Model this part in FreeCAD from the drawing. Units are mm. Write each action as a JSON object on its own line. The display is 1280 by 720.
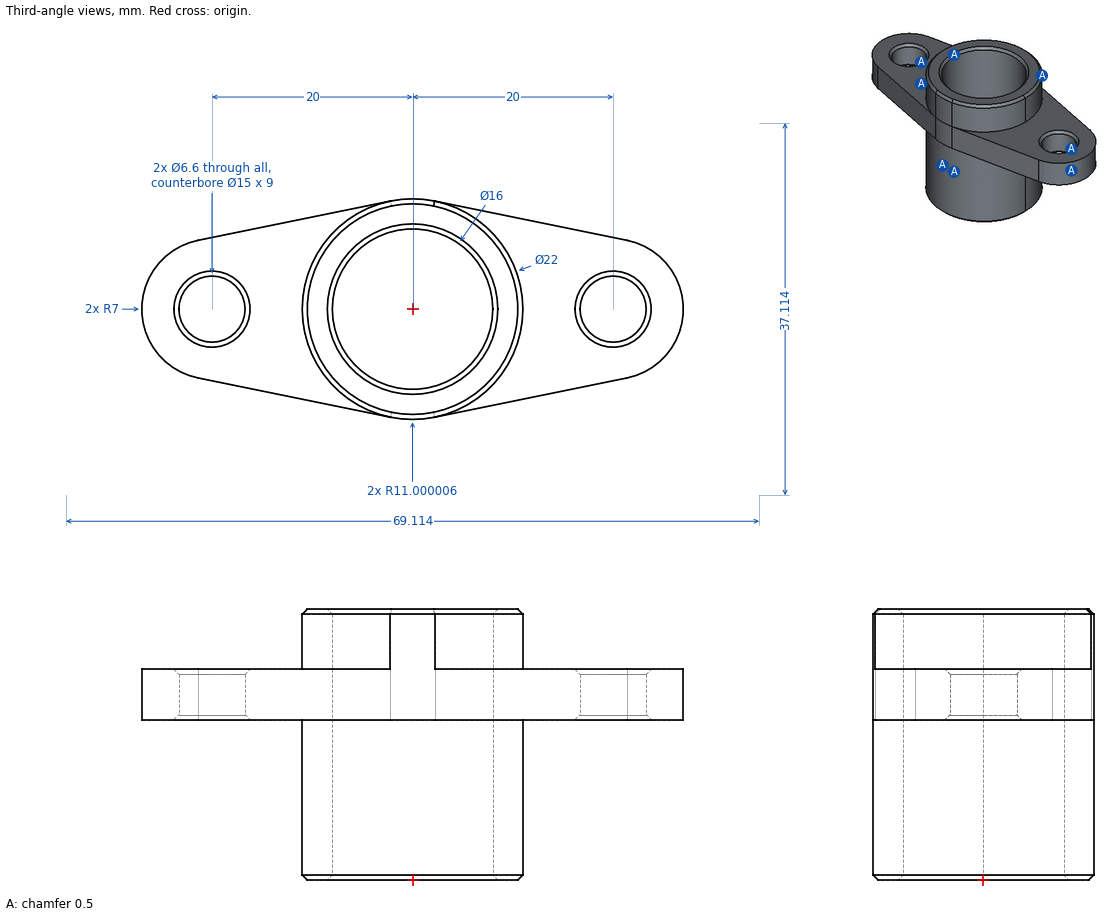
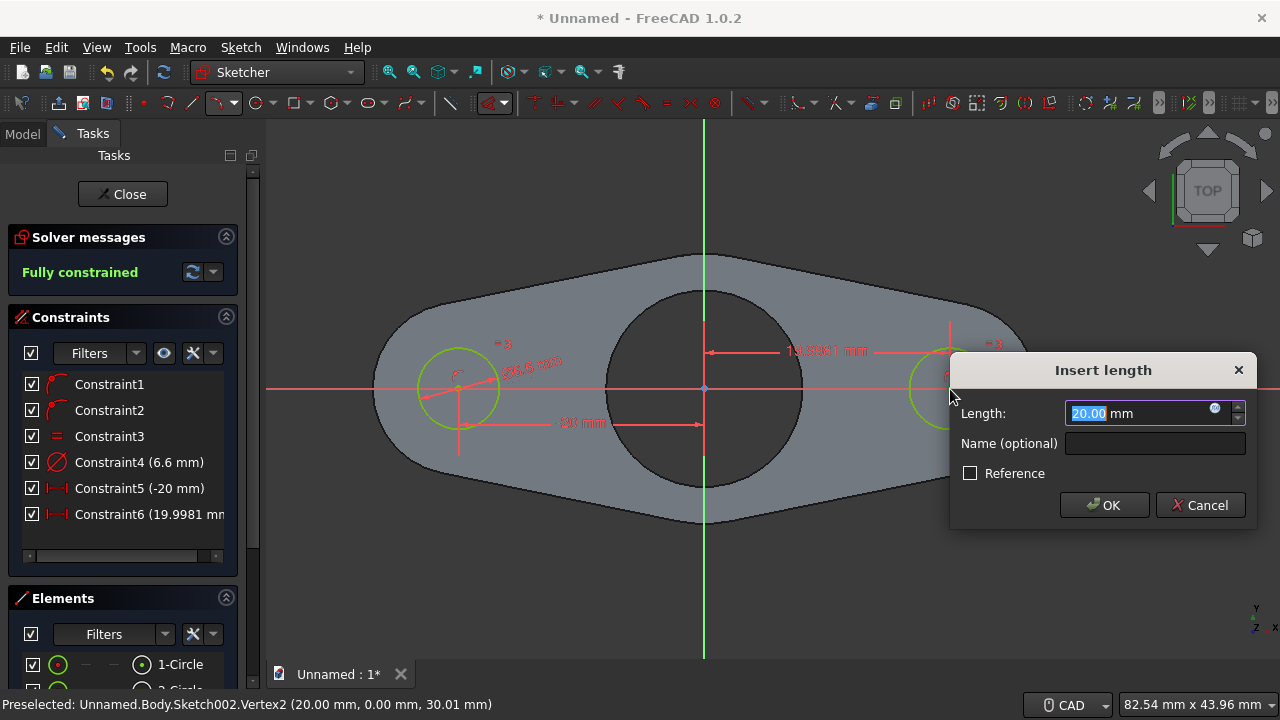
{"action": "type", "text": "20"}
{"action": "key", "text": "Return"}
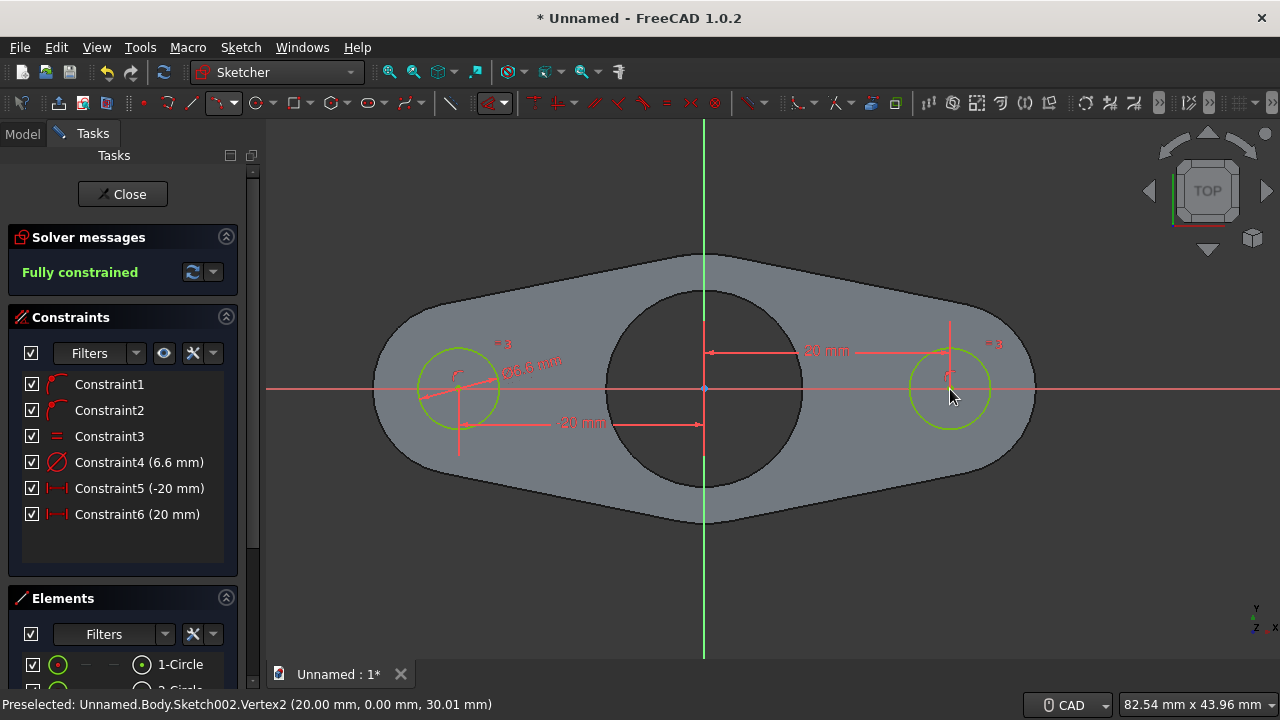
{"action": "left_click", "coordinate": [123, 194]}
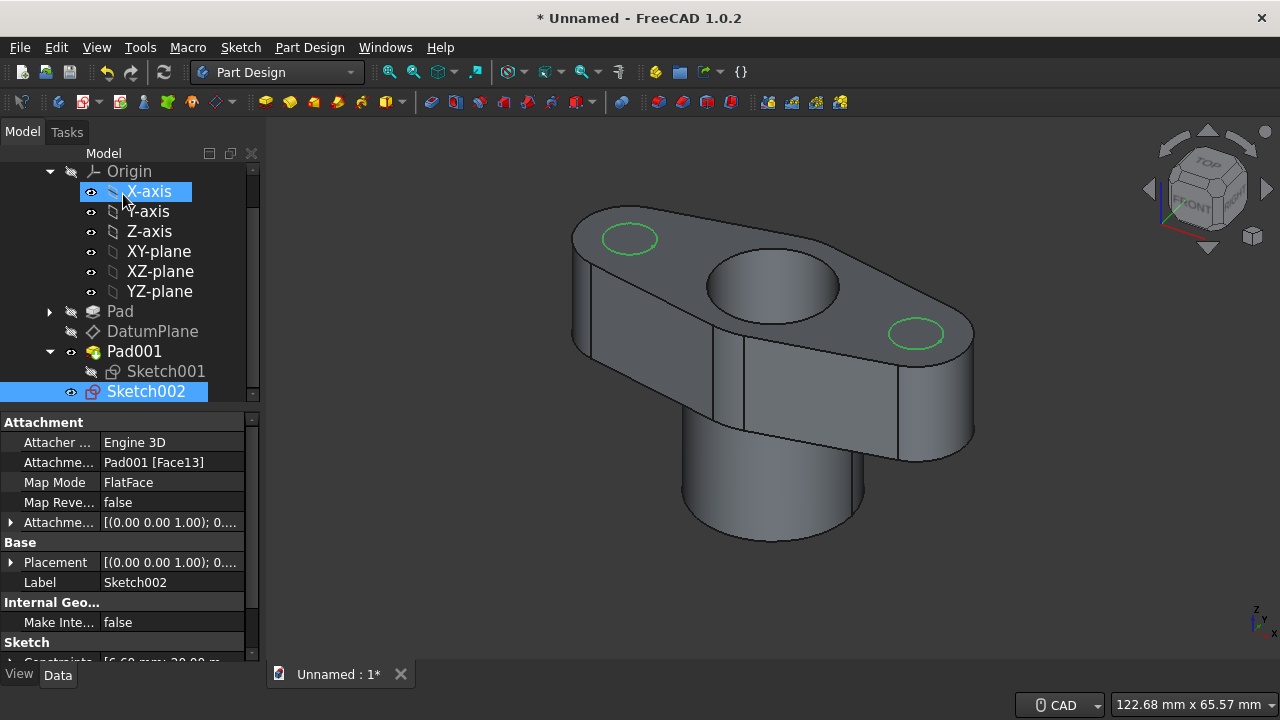
{"action": "left_click", "coordinate": [456, 102]}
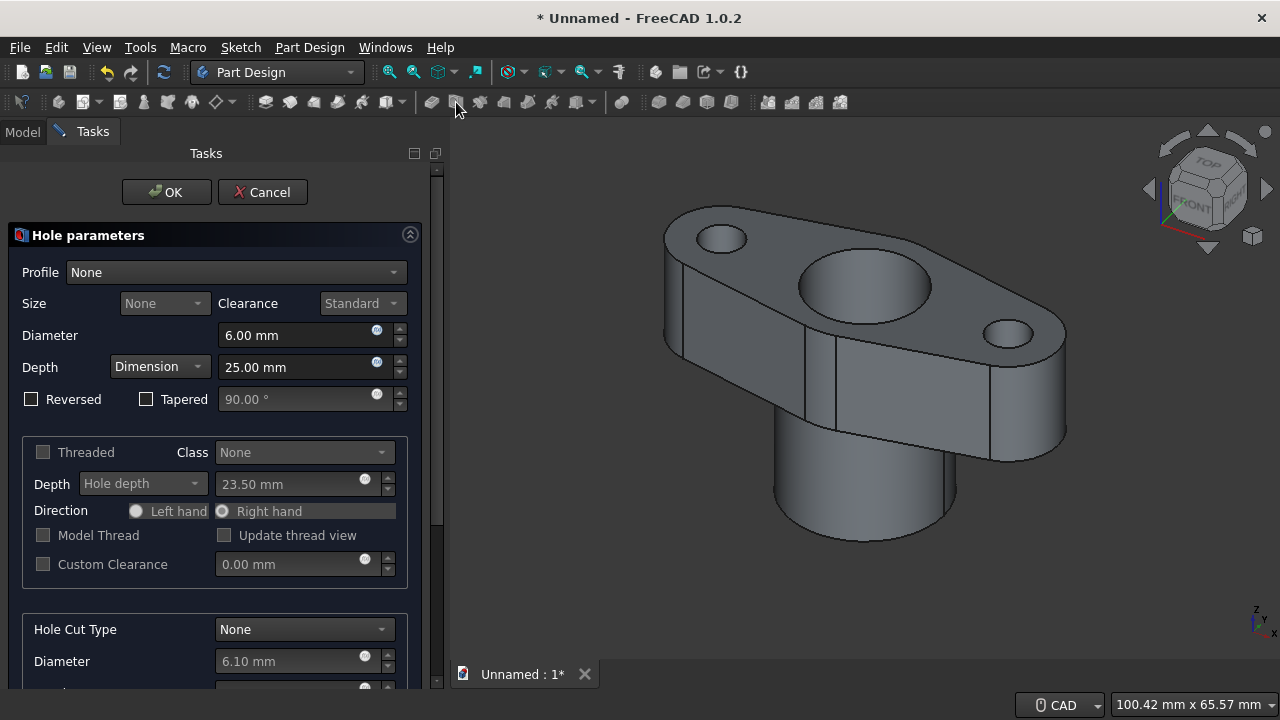
{"action": "triple_click", "coordinate": [305, 335]}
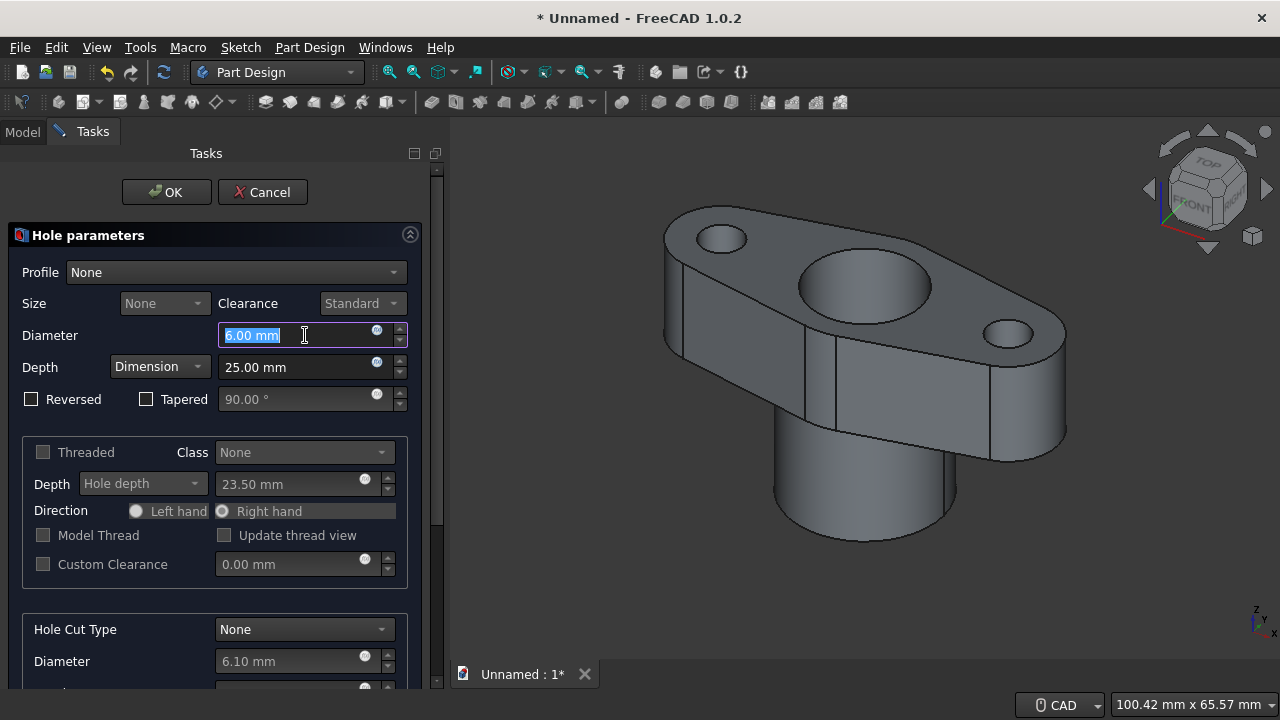
{"action": "type", "text": "6.6"}
{"action": "key", "text": "Tab"}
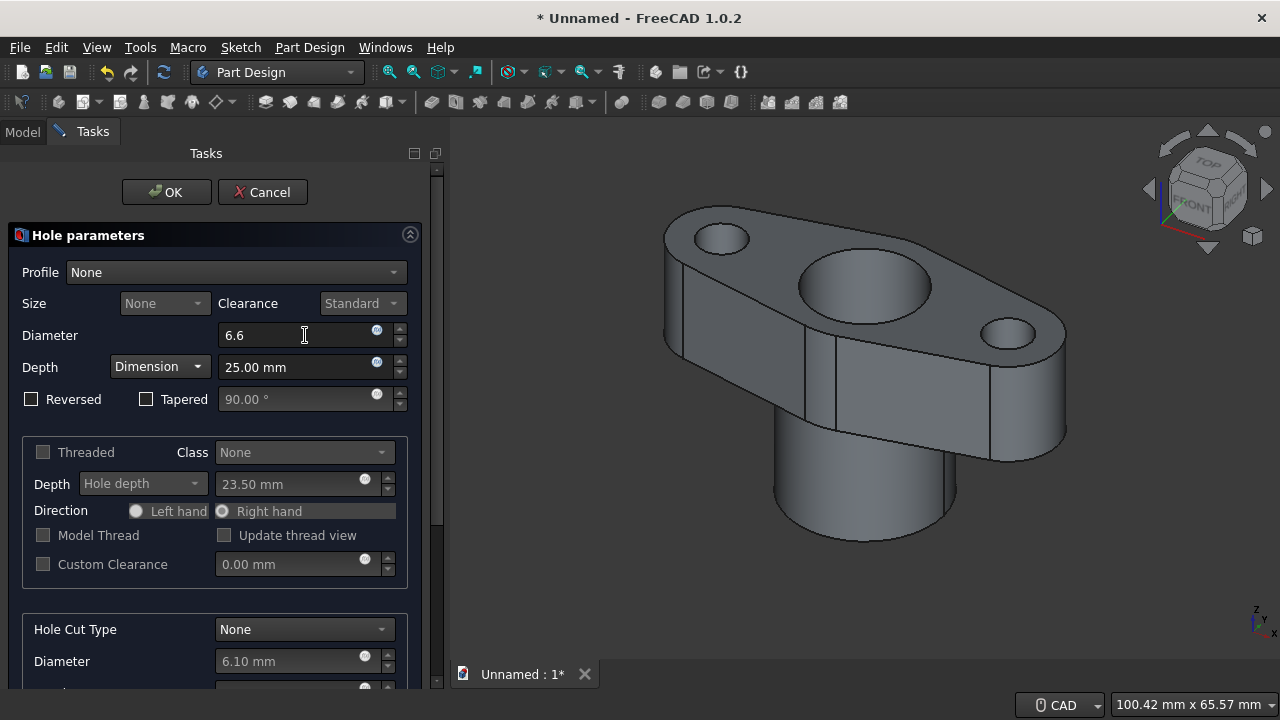
{"action": "left_click", "coordinate": [161, 366]}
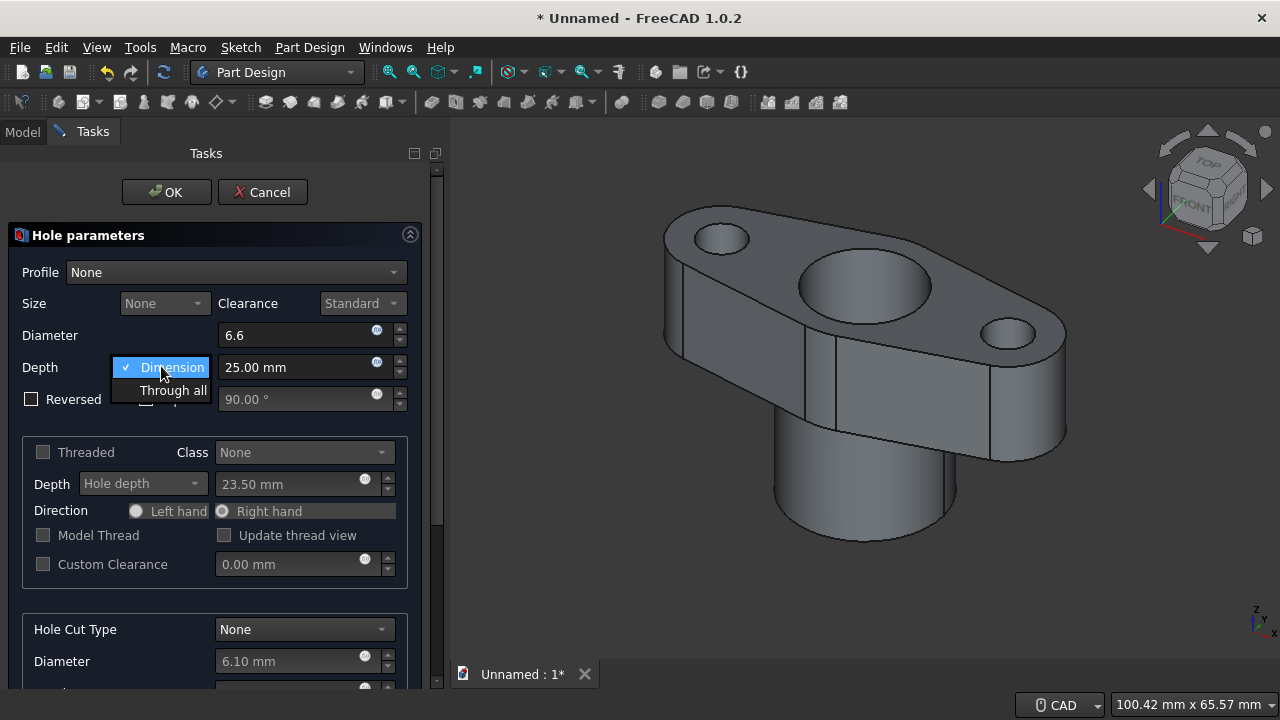
{"action": "left_click", "coordinate": [160, 390]}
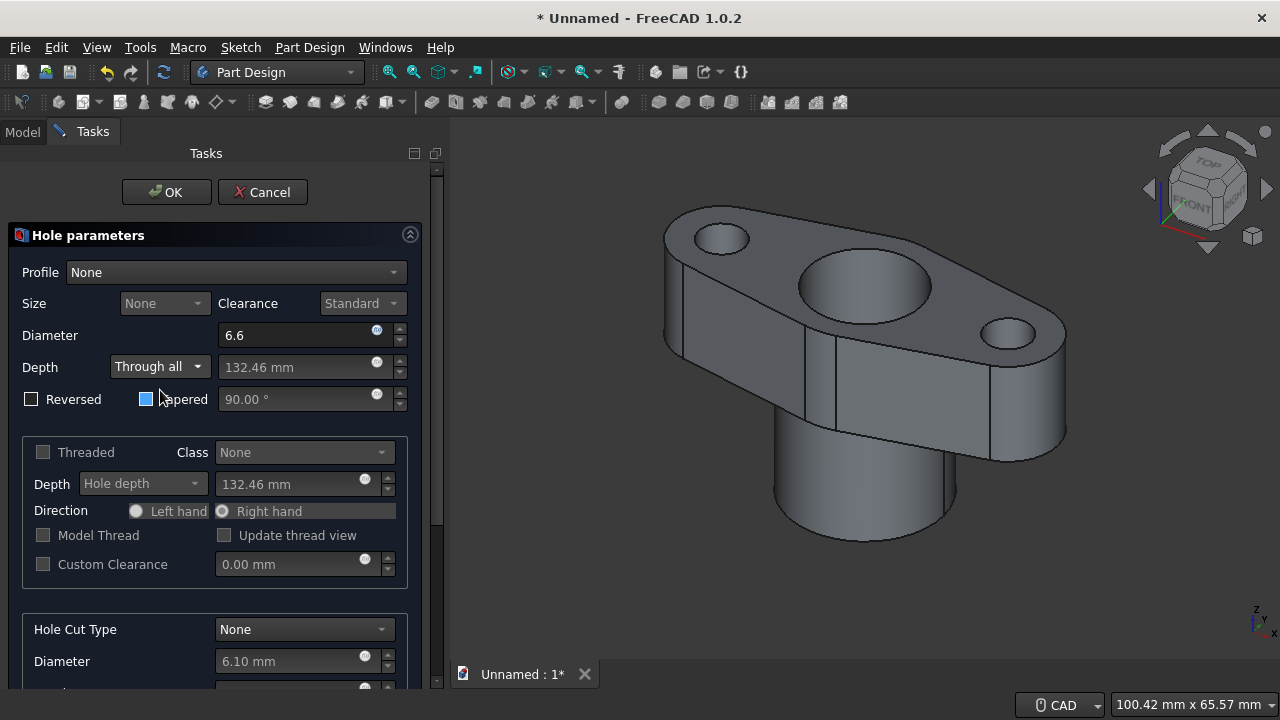
{"action": "left_click", "coordinate": [306, 630]}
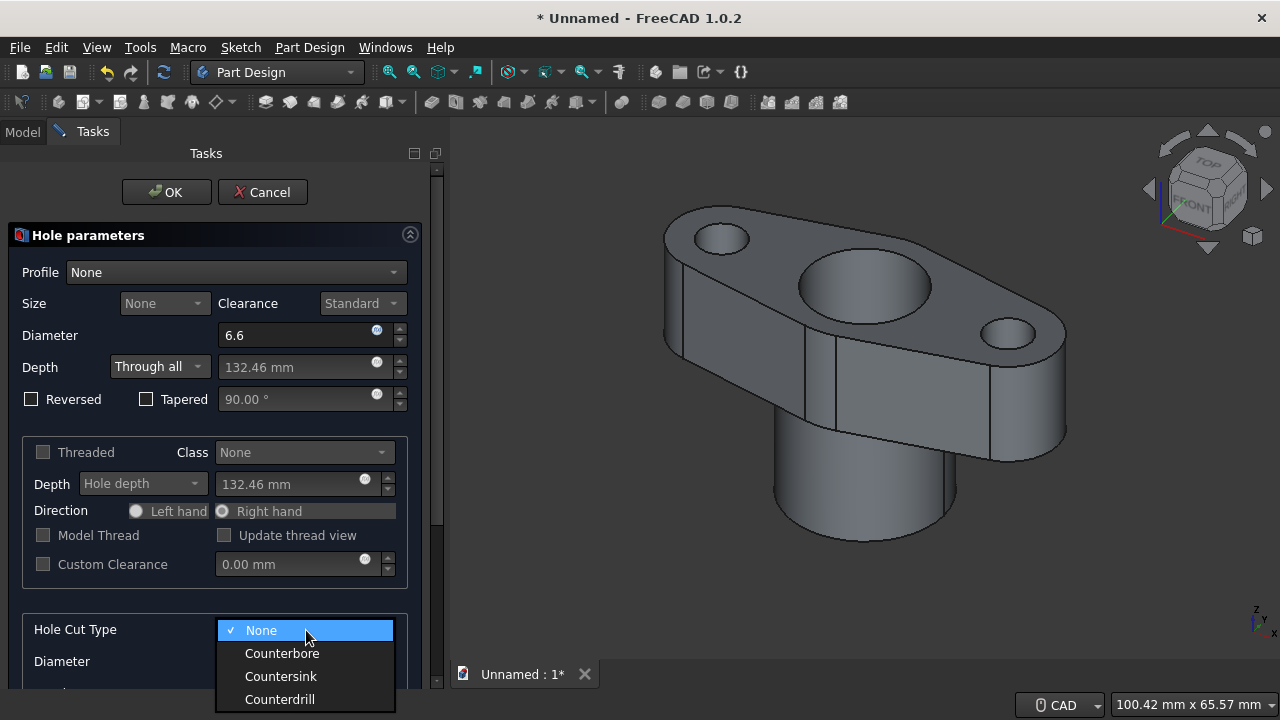
{"action": "left_click", "coordinate": [304, 654]}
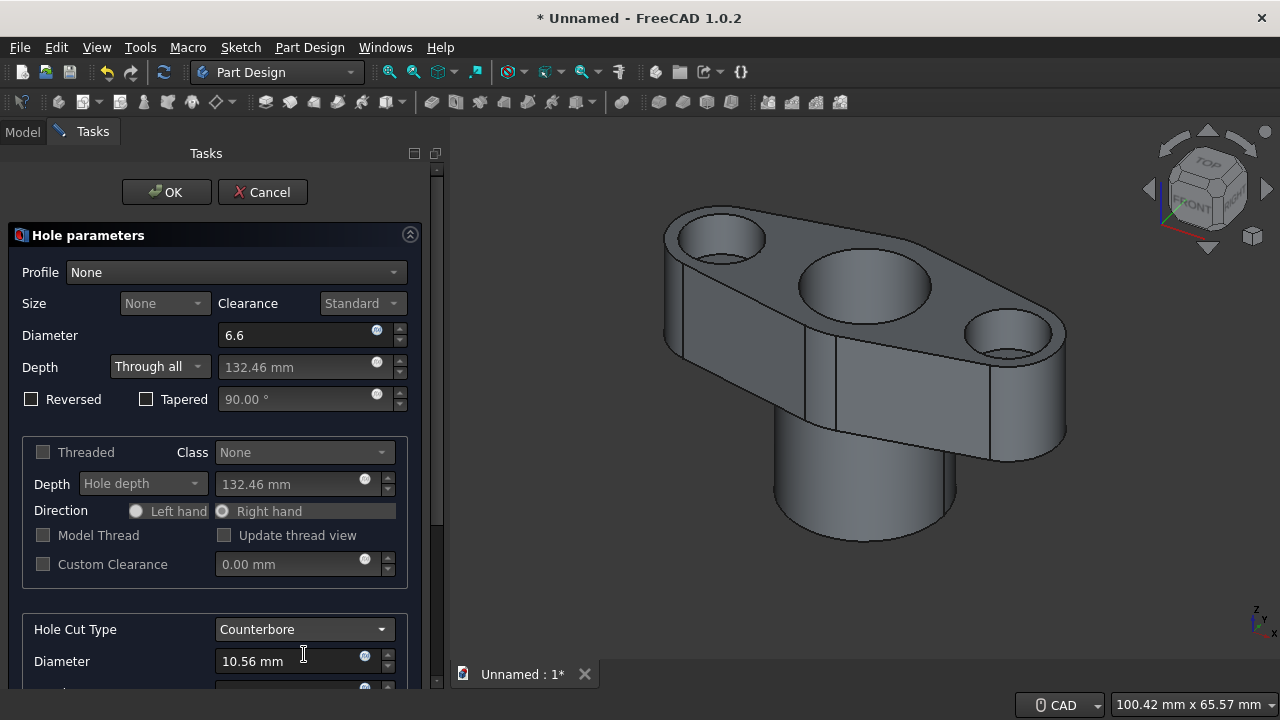
{"action": "triple_click", "coordinate": [298, 661]}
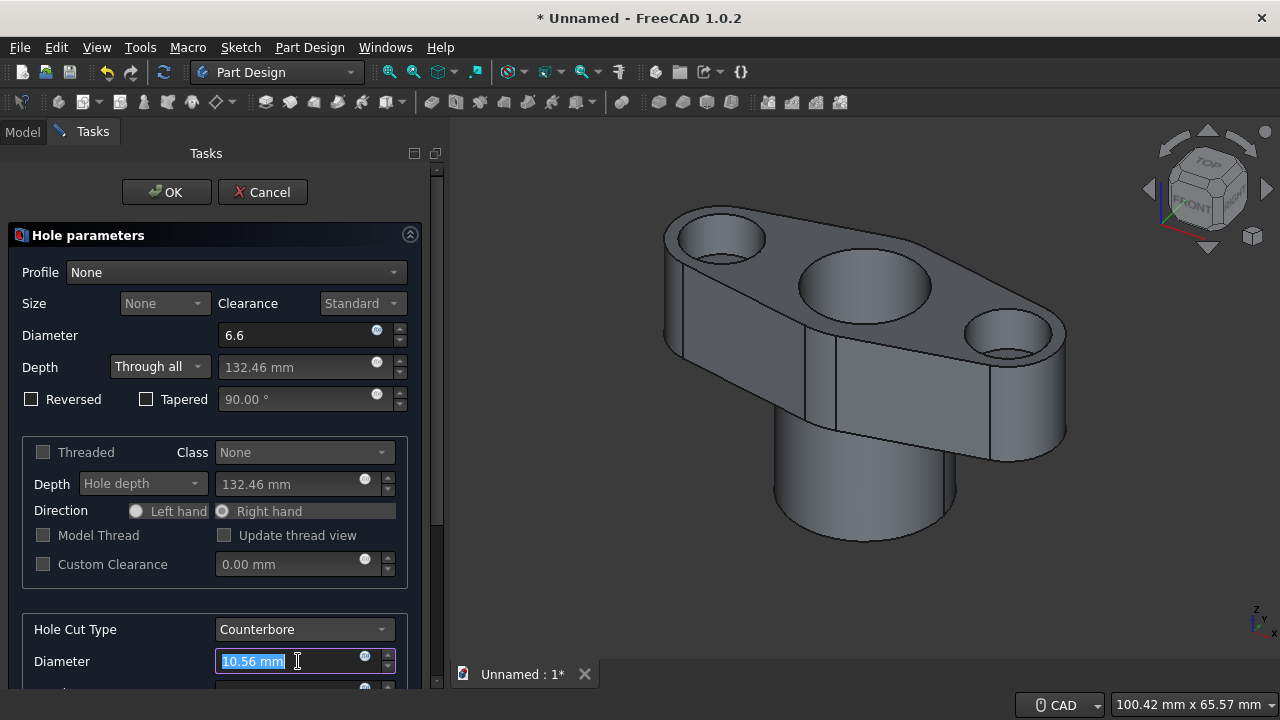
{"action": "type", "text": "15"}
{"action": "key", "text": "Tab"}